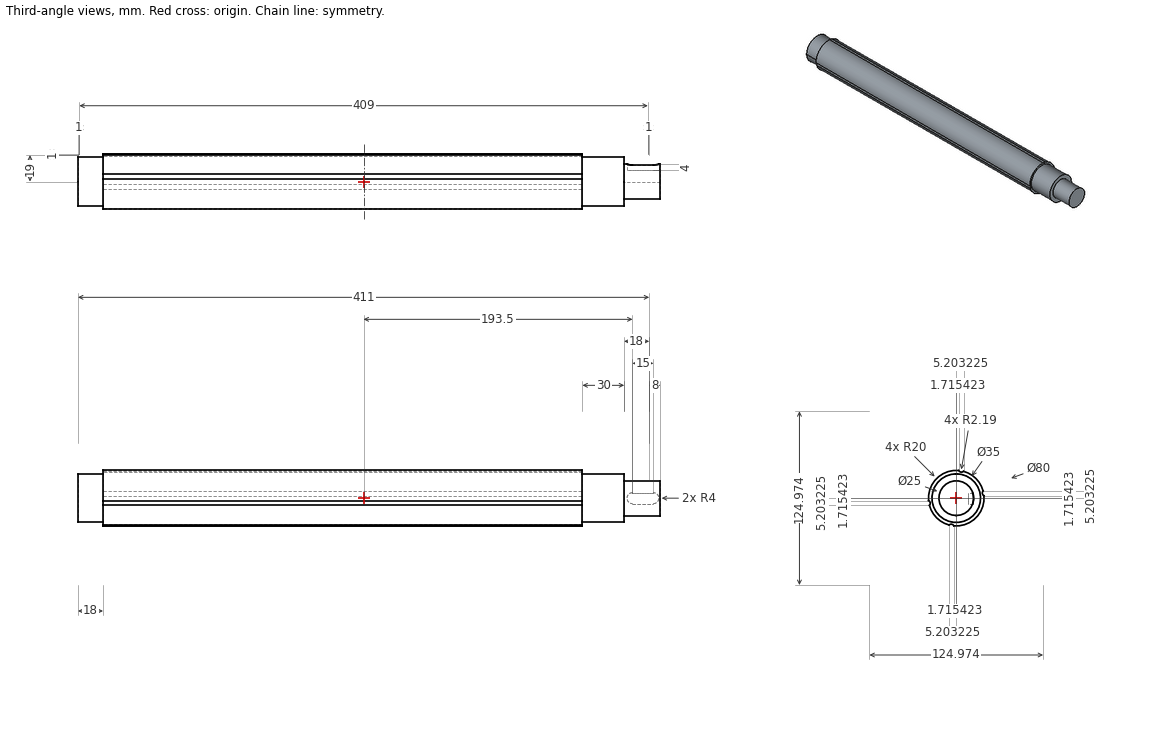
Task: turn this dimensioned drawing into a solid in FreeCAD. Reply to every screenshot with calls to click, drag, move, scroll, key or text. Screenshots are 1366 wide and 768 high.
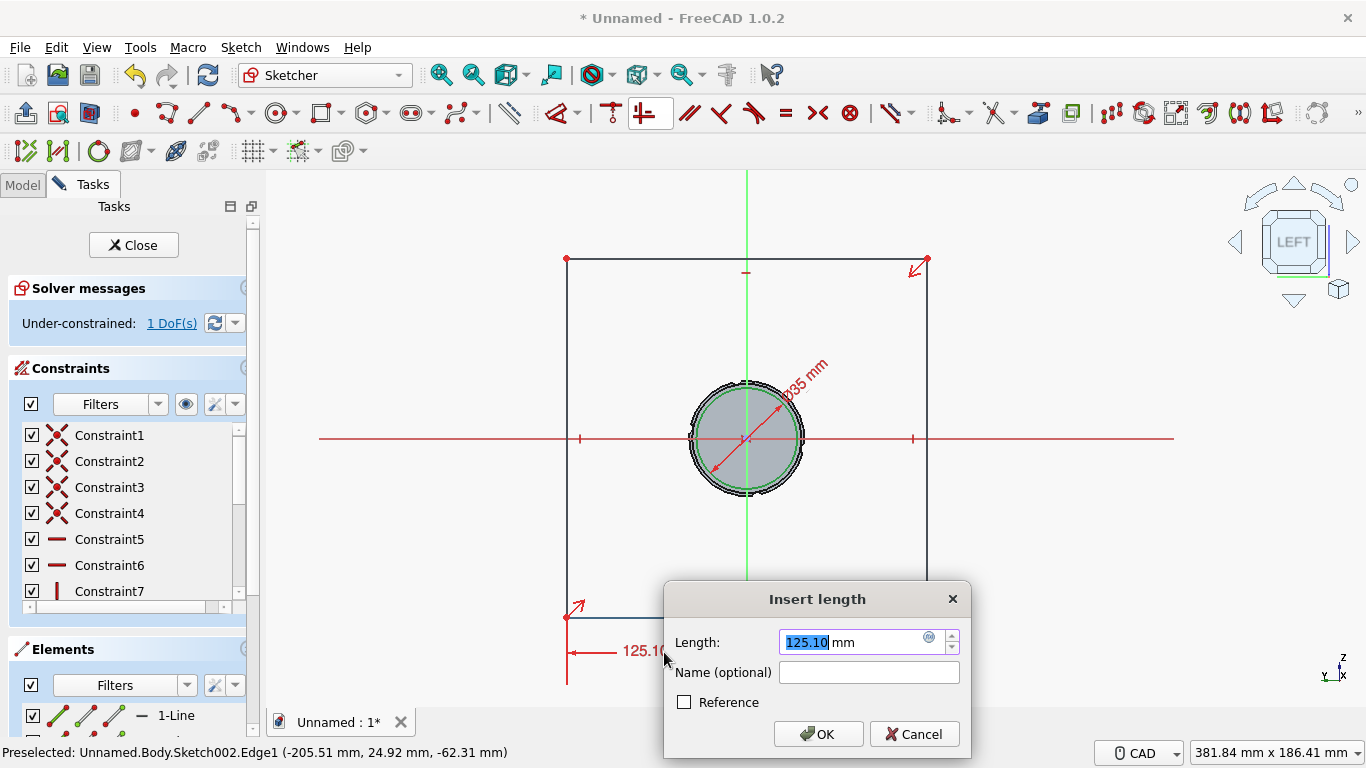
text(124.974)
key(Return)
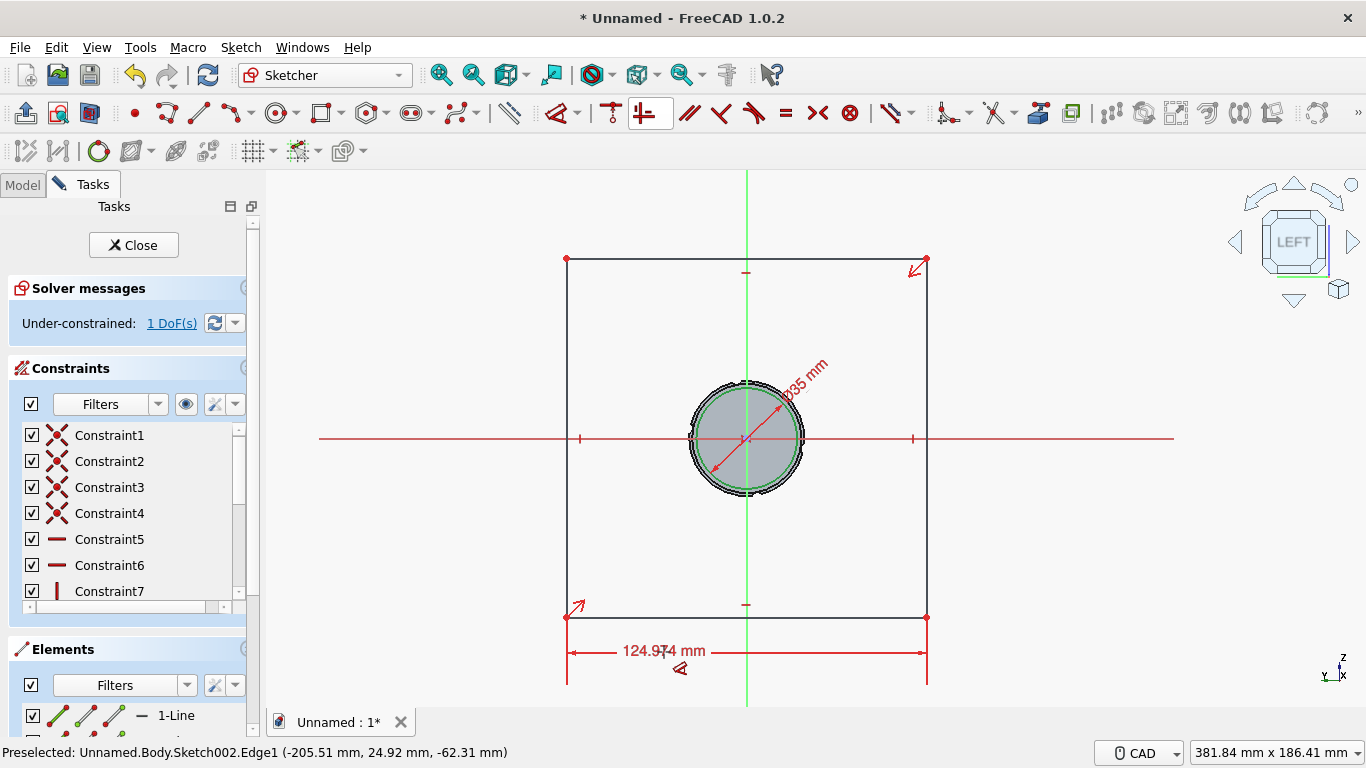
click(927, 510)
click(961, 356)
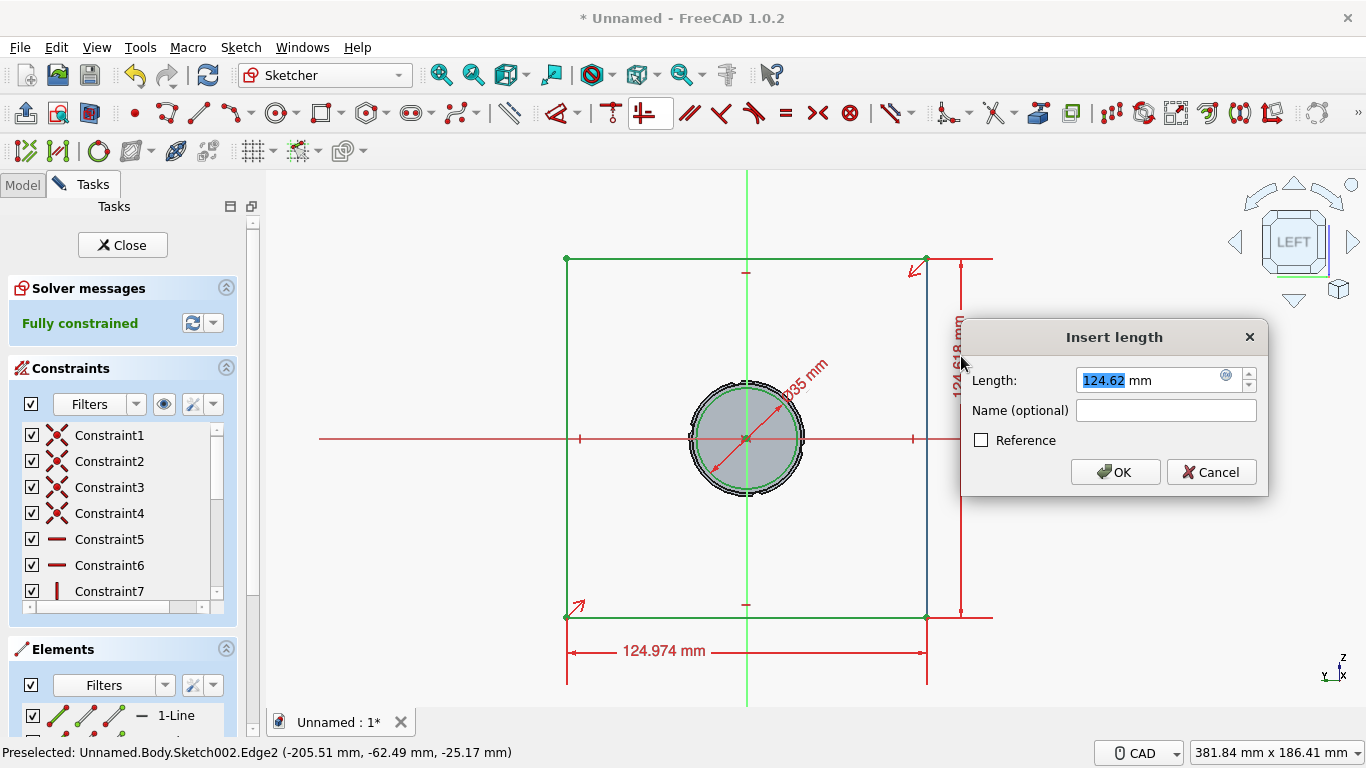
text(124.974)
key(Return)
key(Escape)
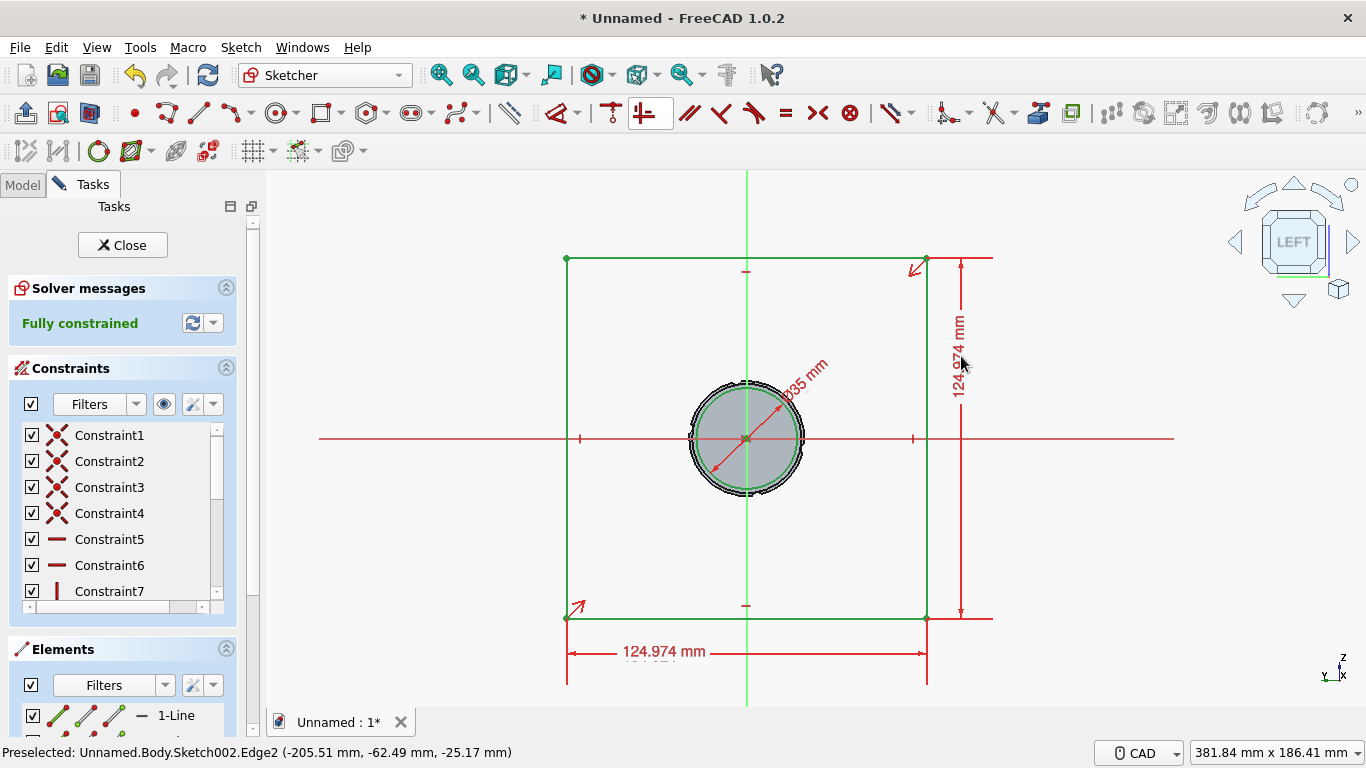
click(123, 245)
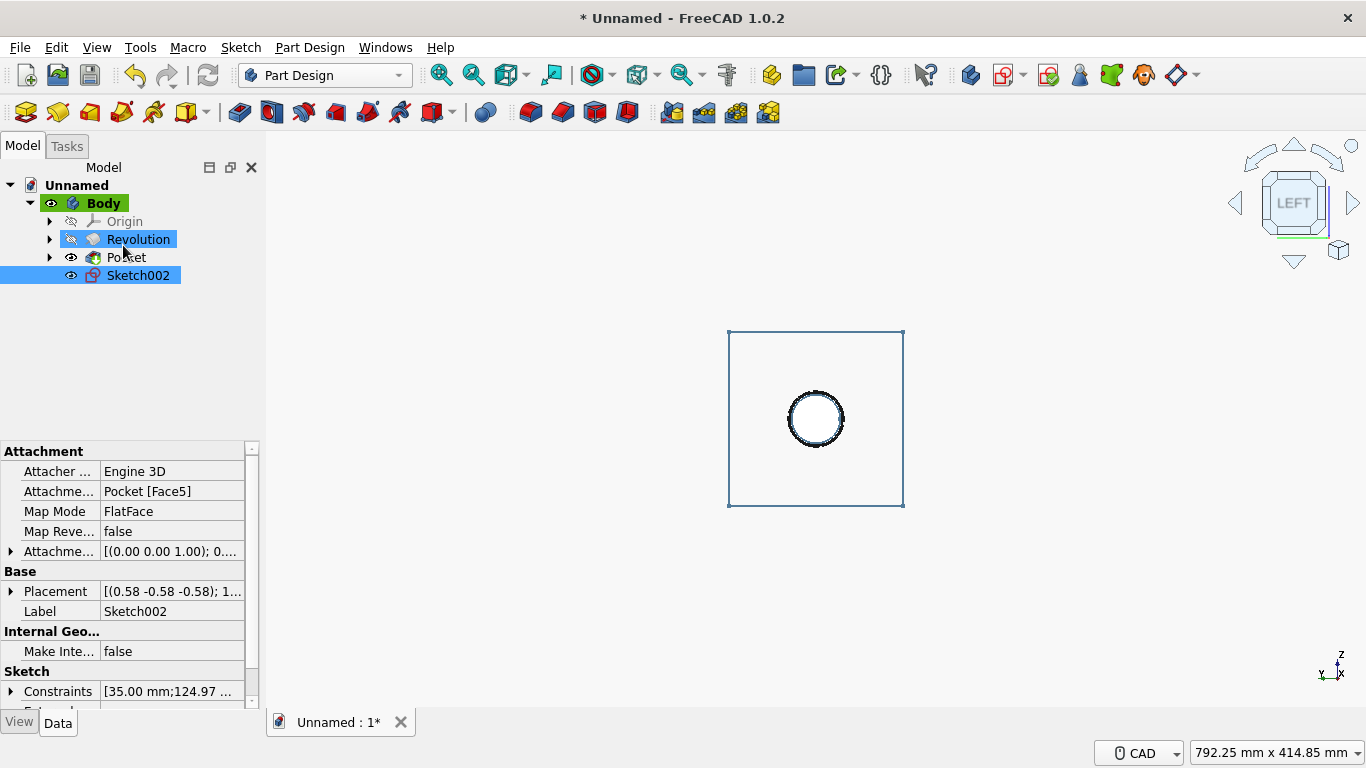
click(240, 112)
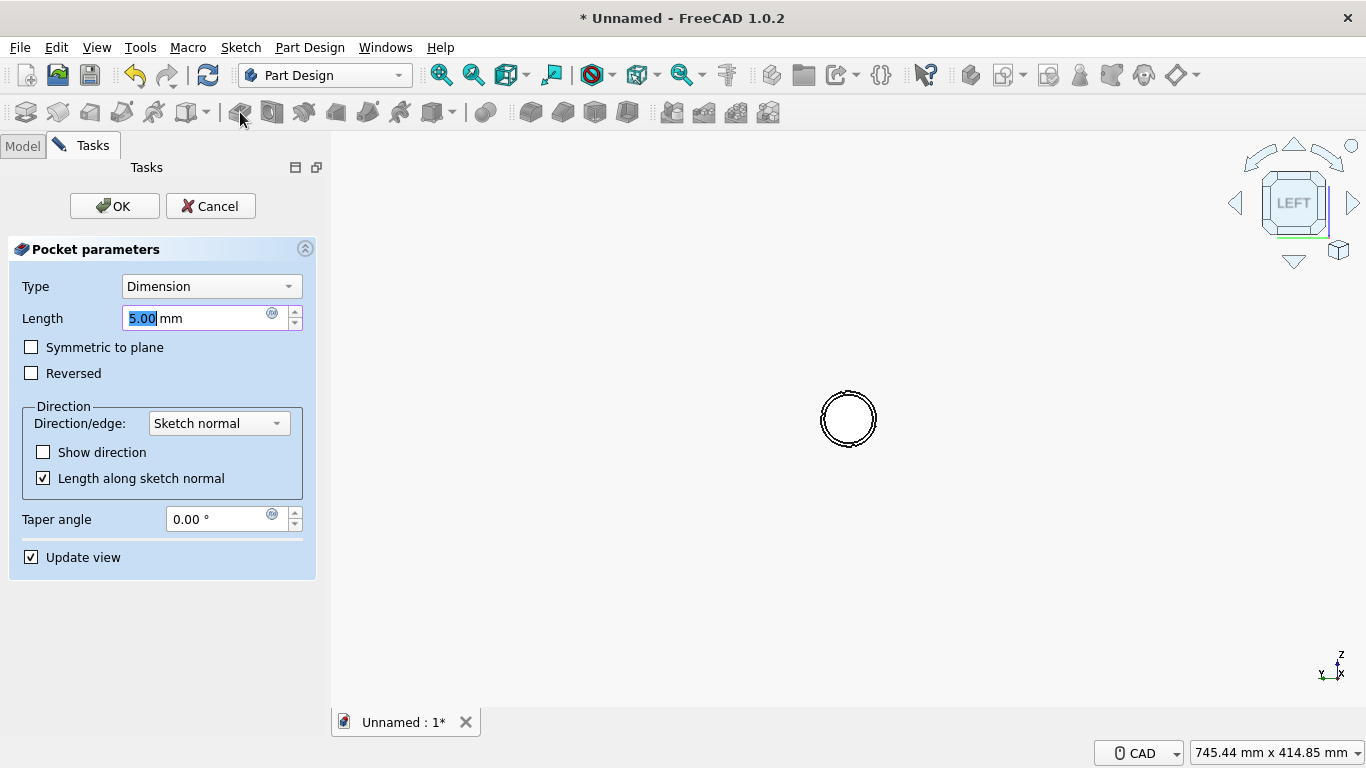
text(18)
key(Tab)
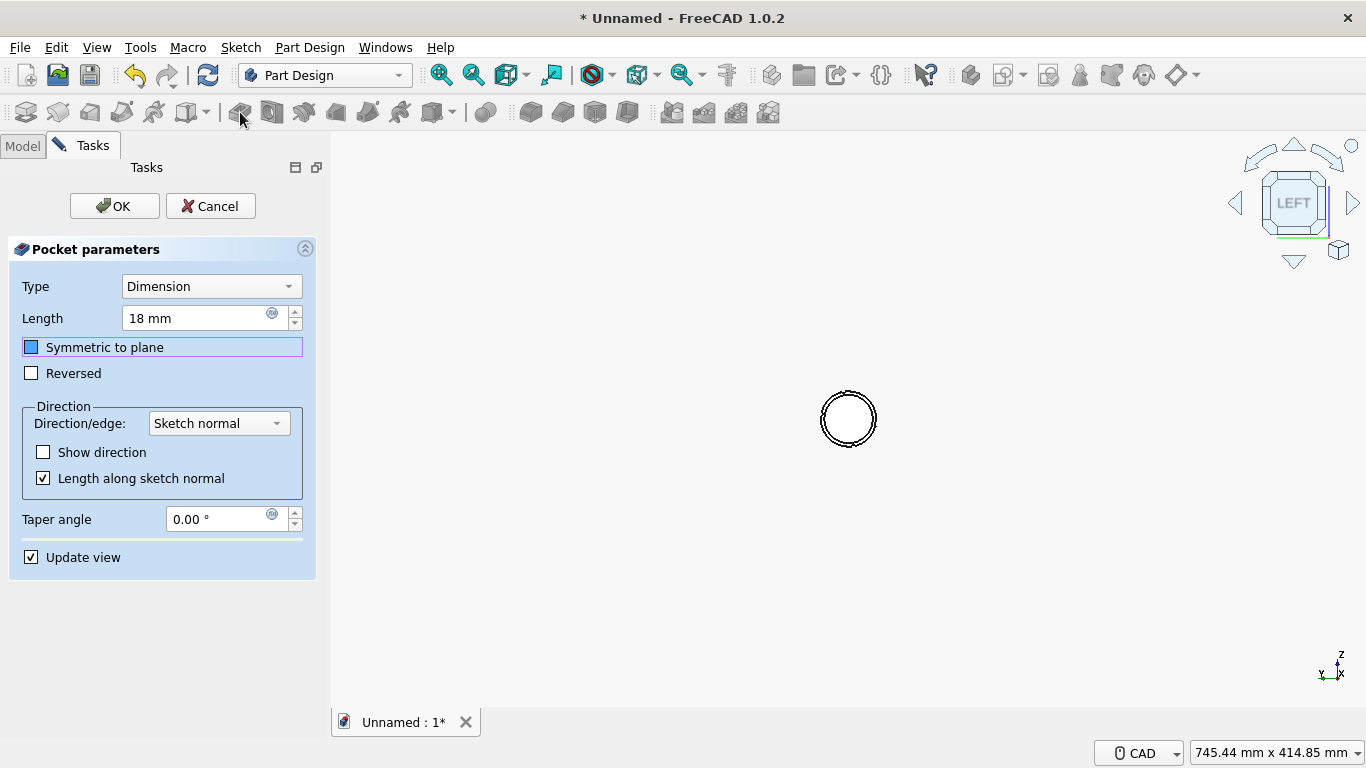
click(115, 206)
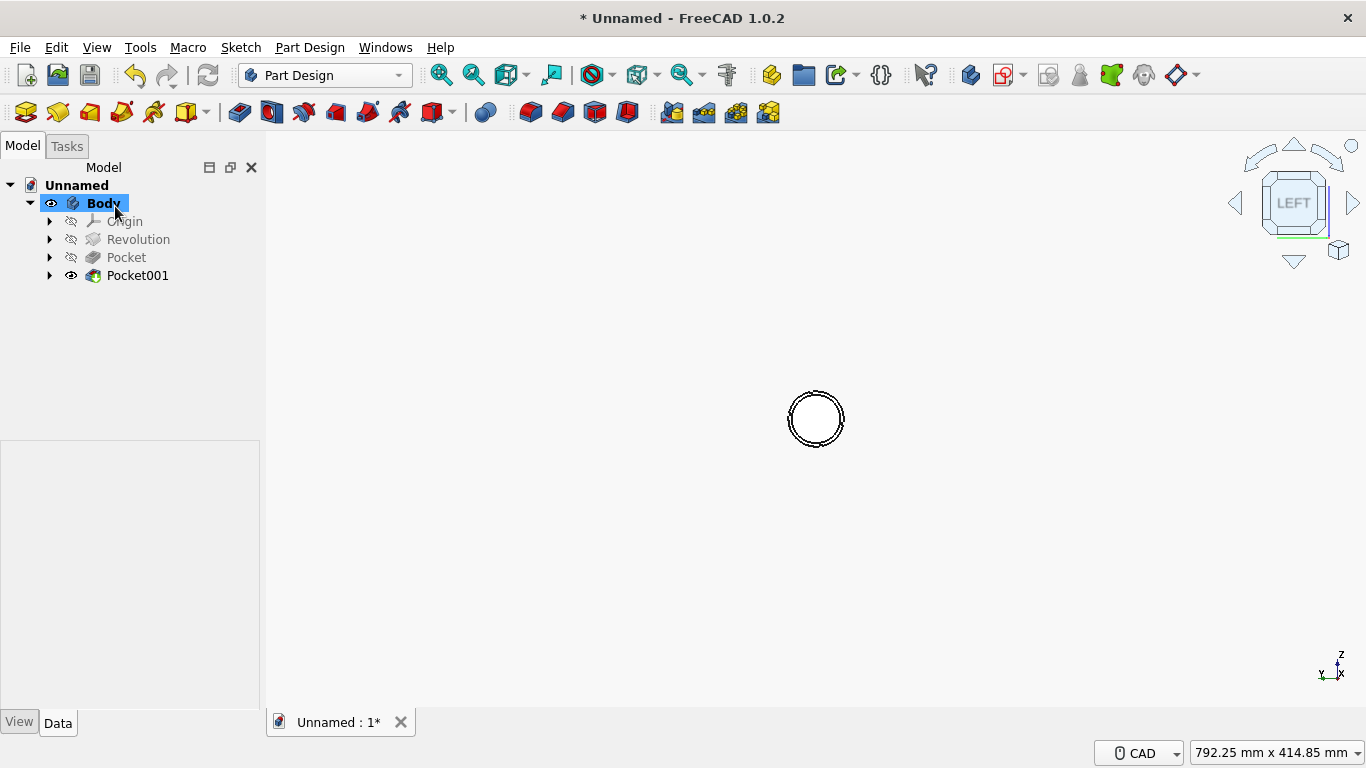
key(v)
key(f)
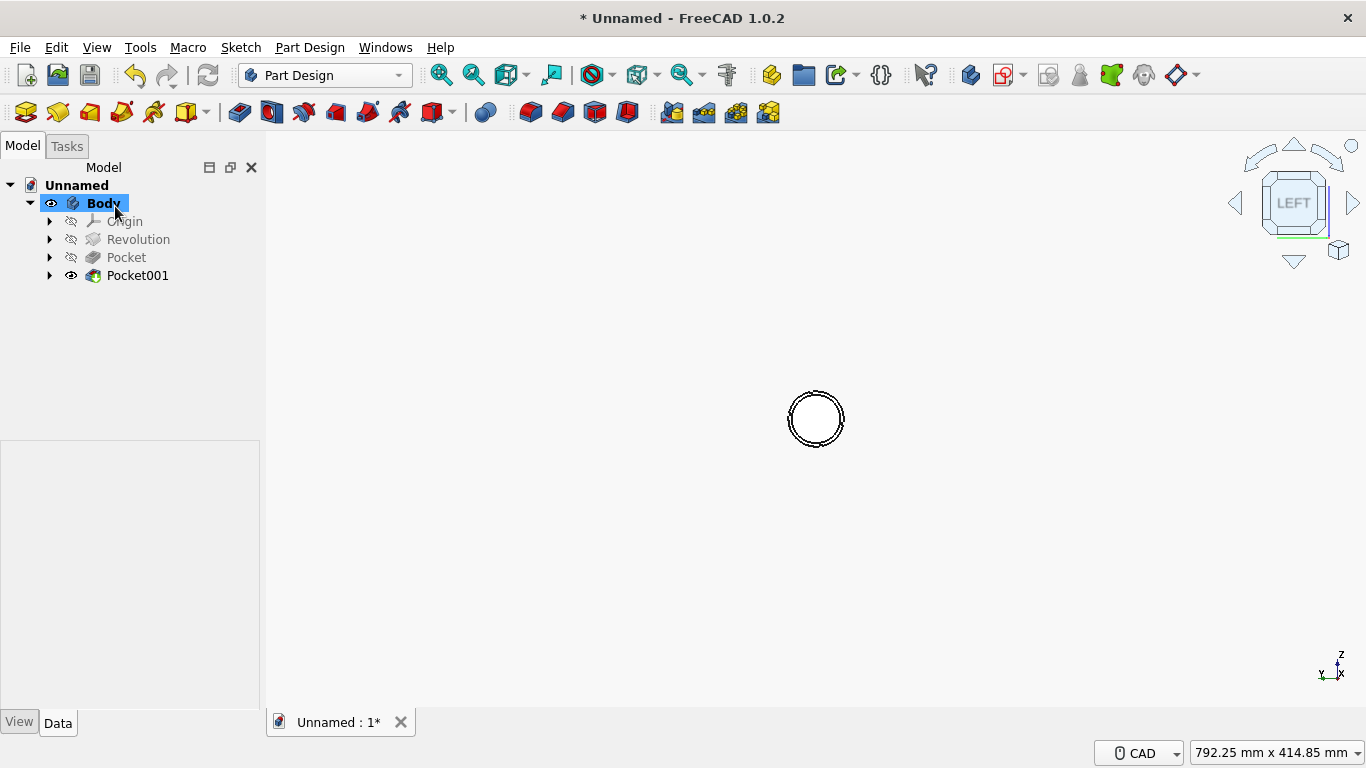
key(0)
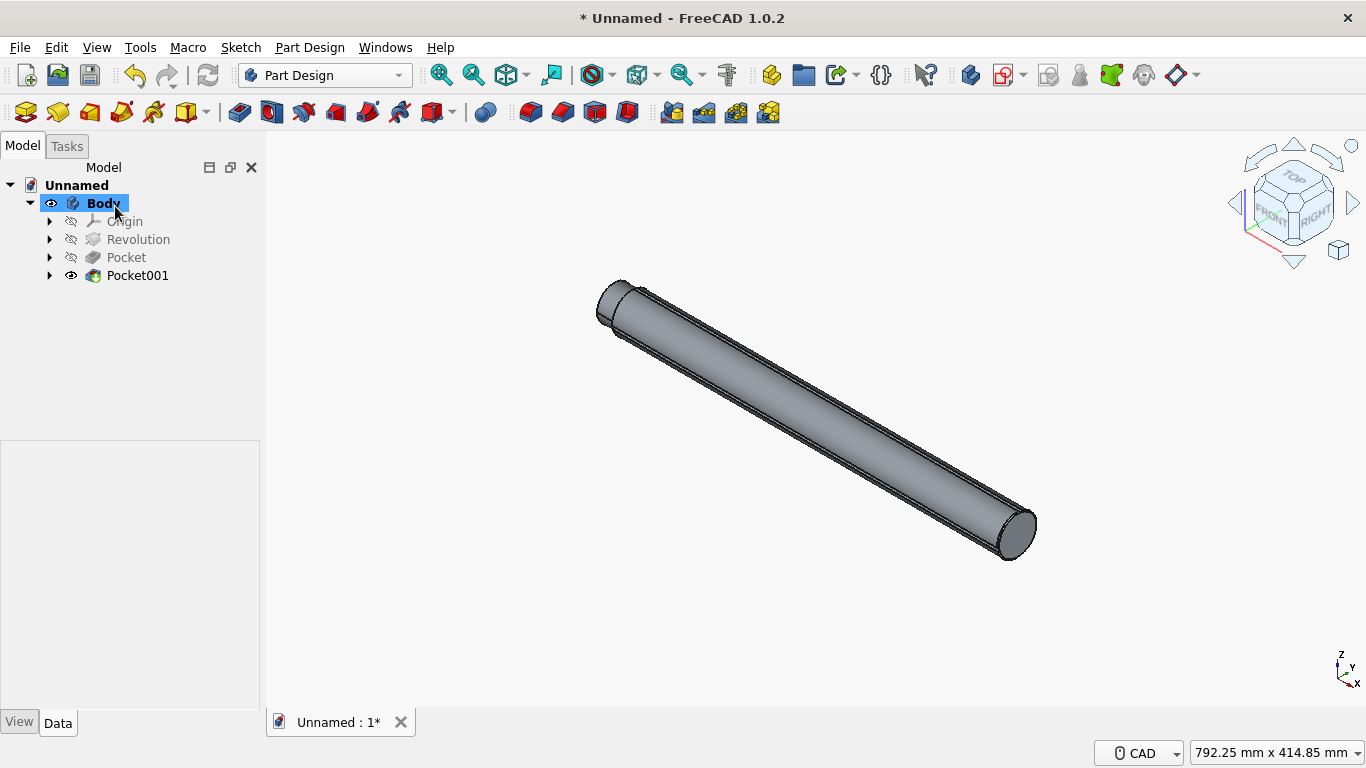
click(1018, 535)